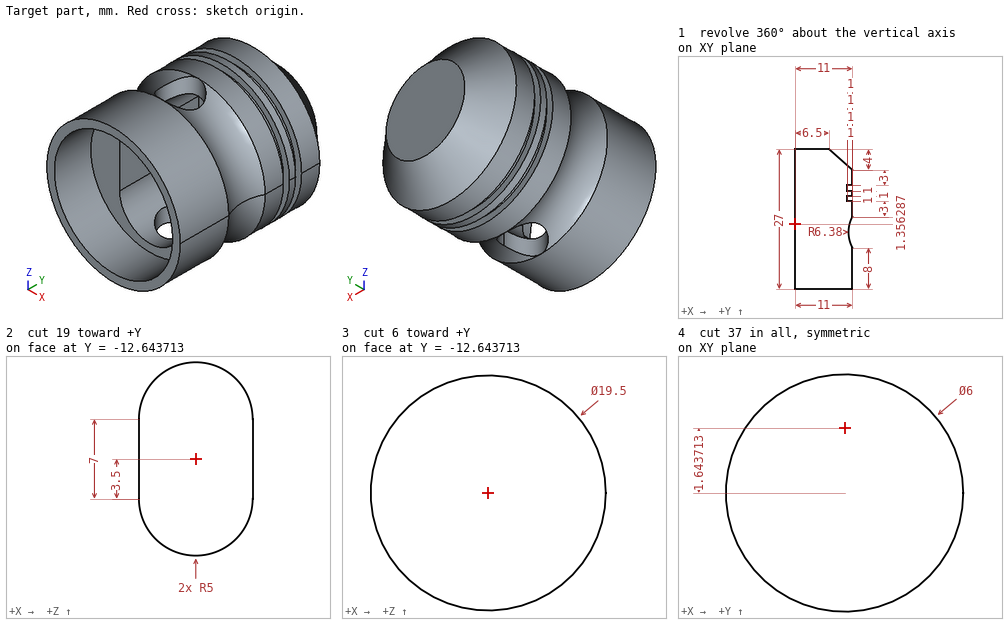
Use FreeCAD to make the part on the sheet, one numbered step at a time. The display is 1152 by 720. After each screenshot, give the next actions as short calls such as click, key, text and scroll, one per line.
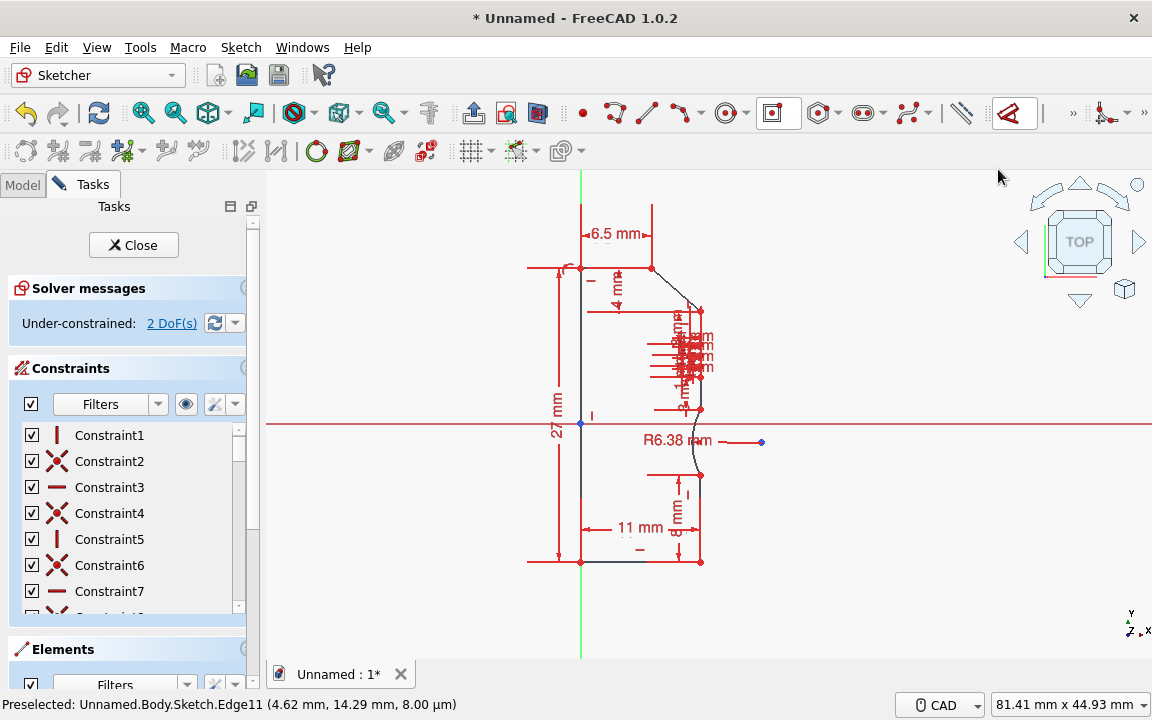
click(701, 410)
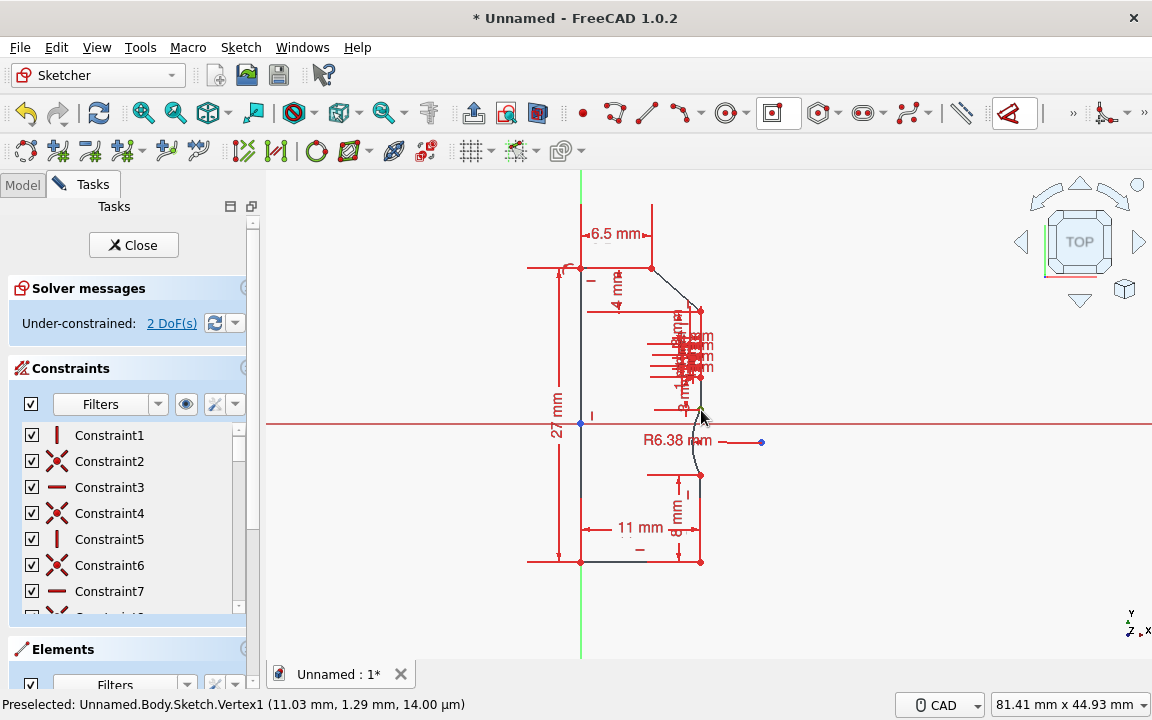
key(l)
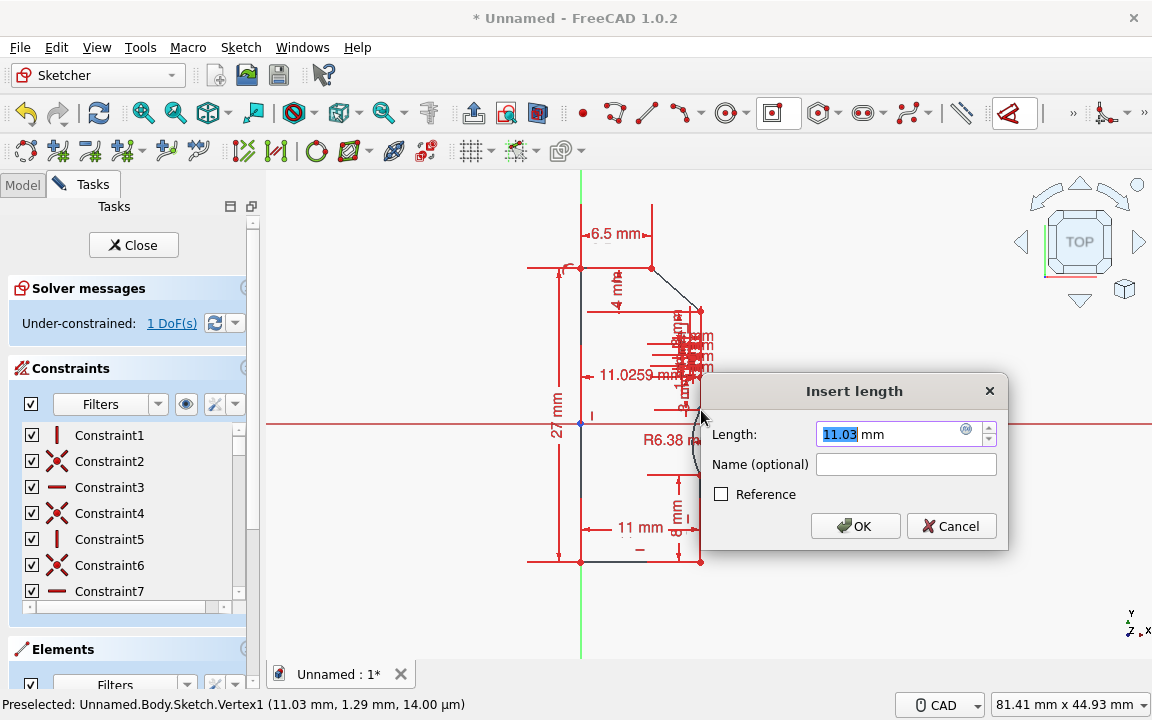
text(11)
key(Return)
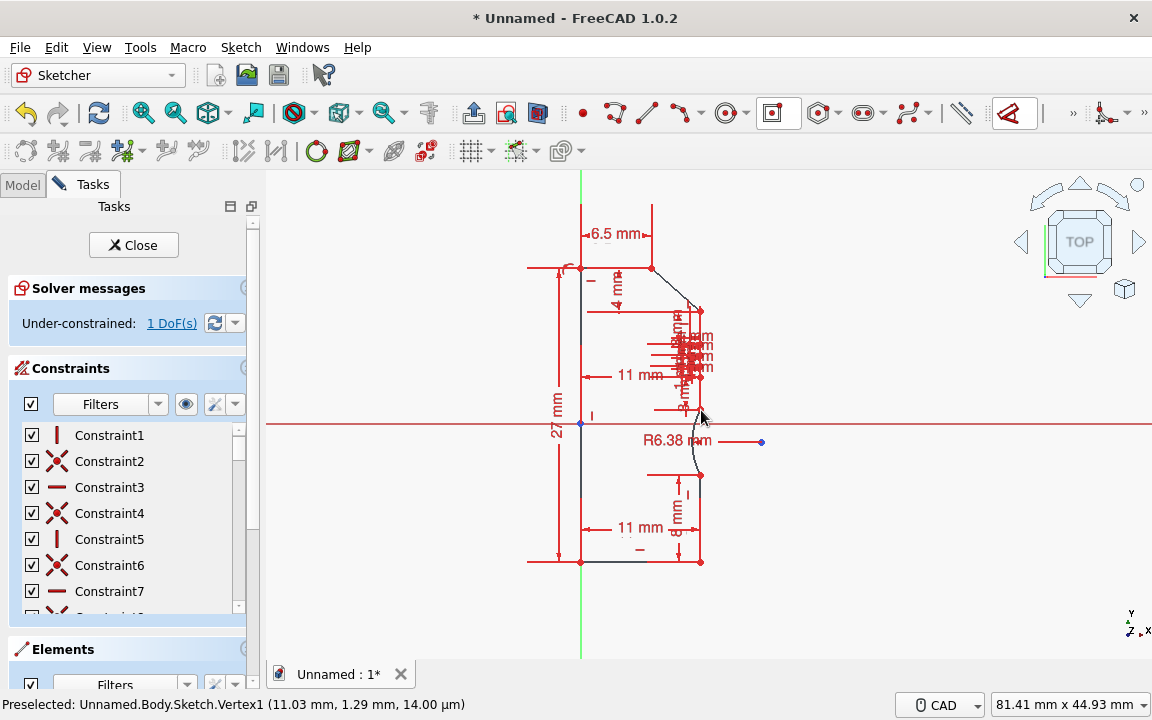
scroll(700, 410, up, 5)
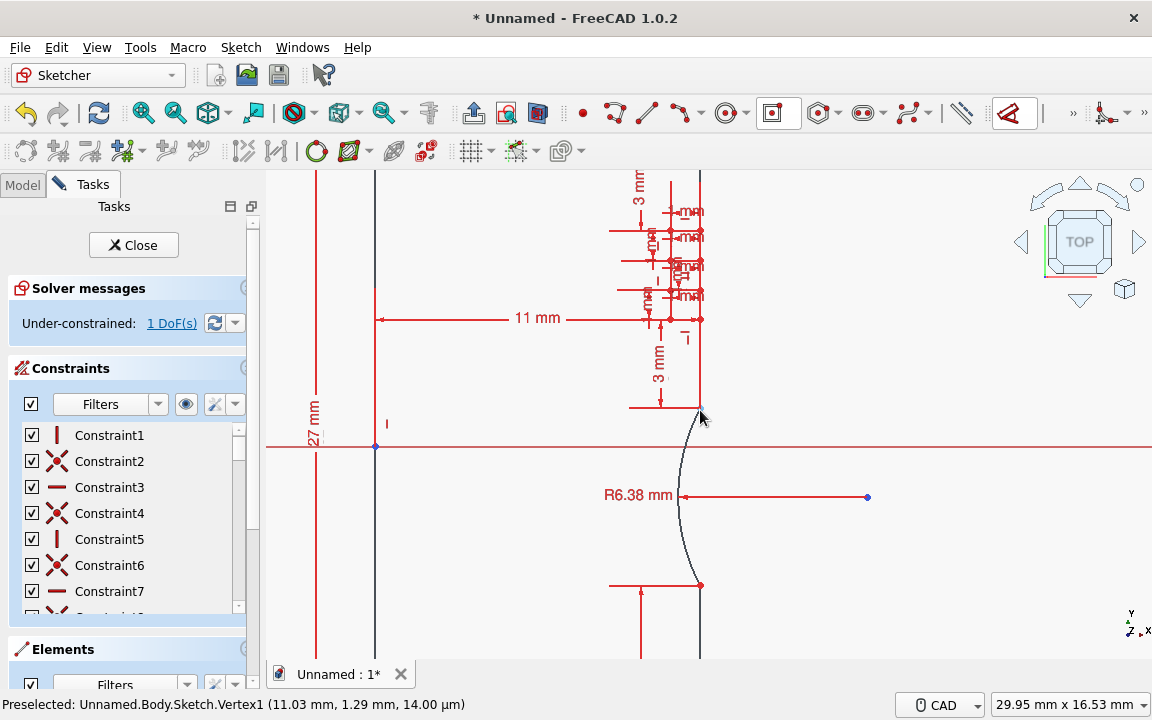
click(700, 408)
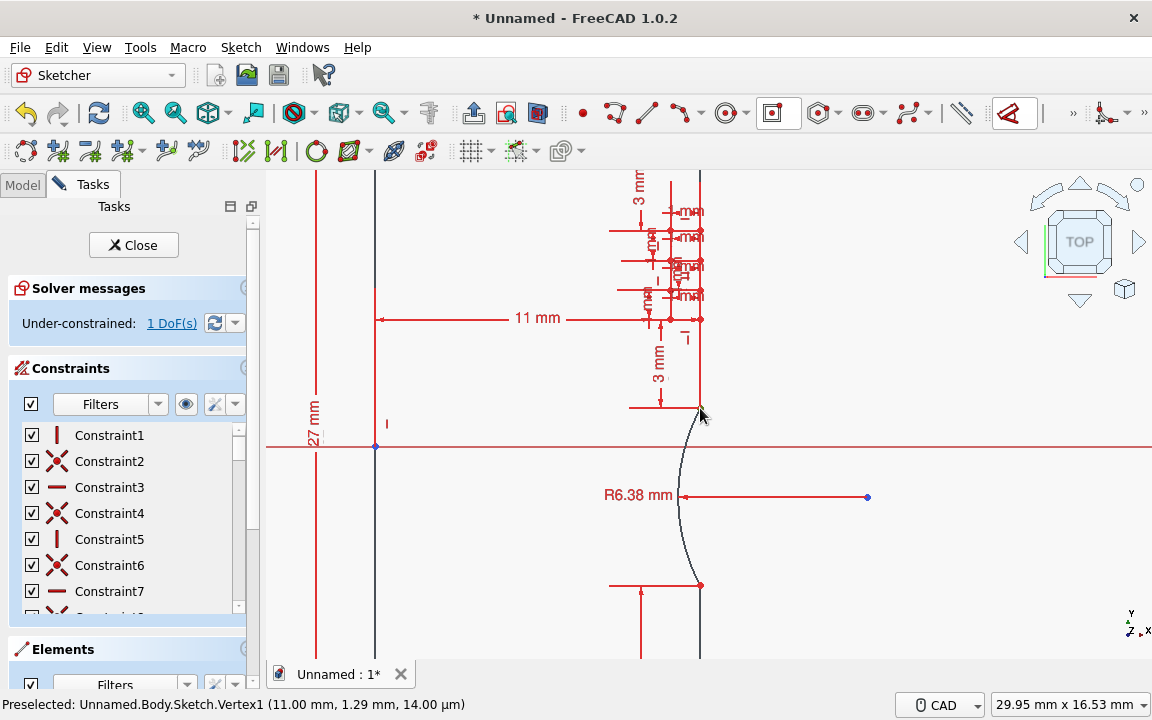
click(1032, 114)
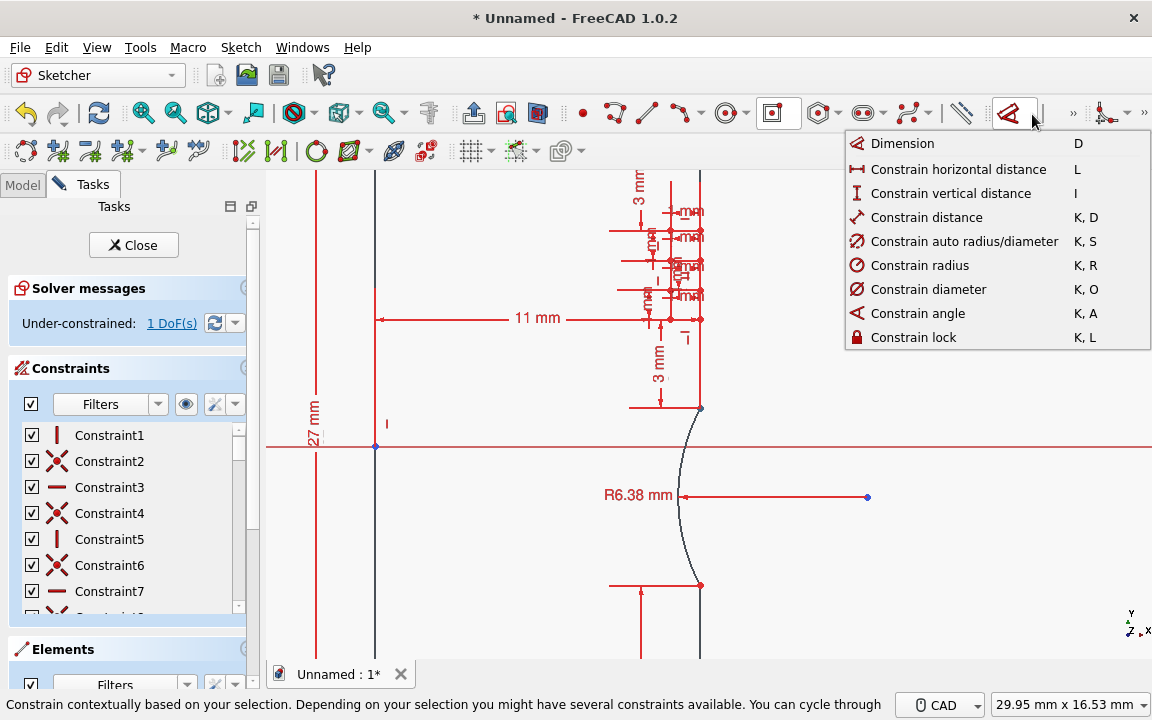
click(998, 193)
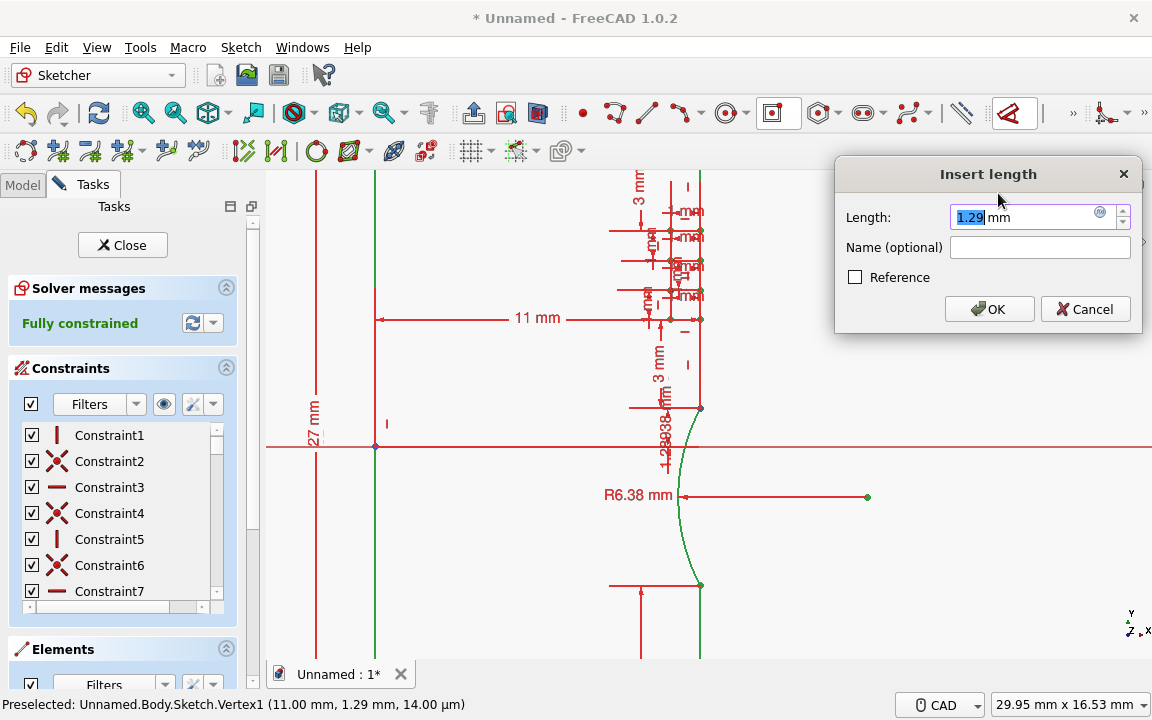
text(1.356287)
key(Return)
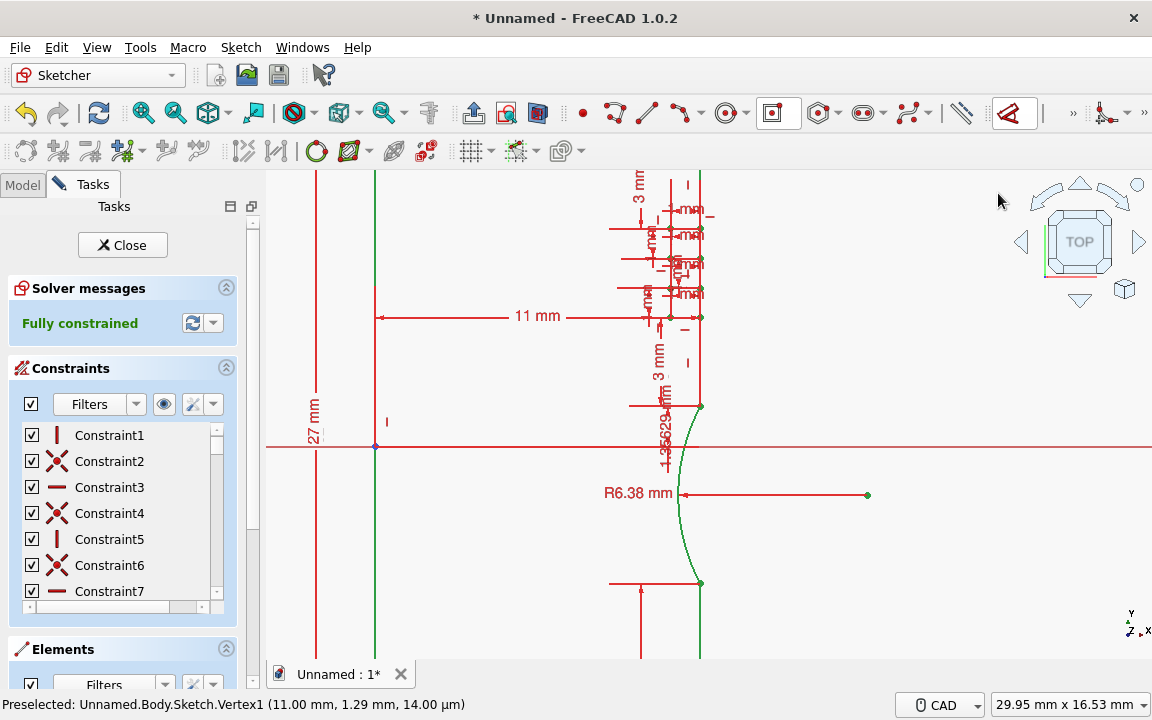
click(123, 245)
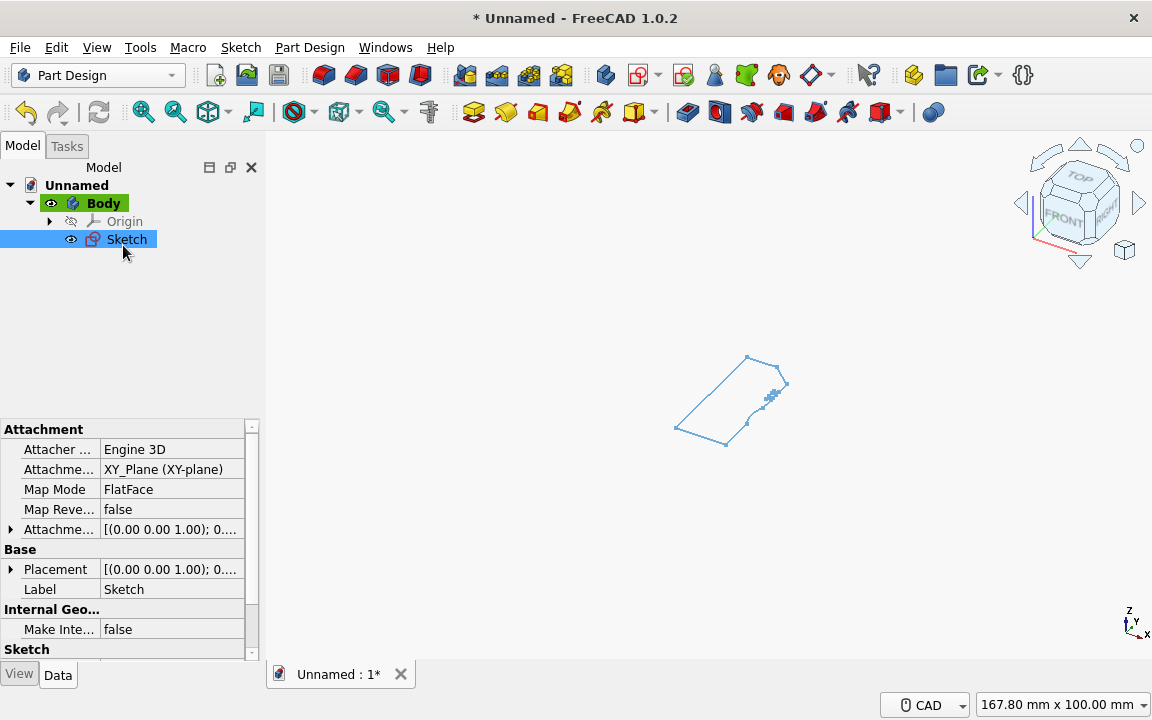
click(506, 112)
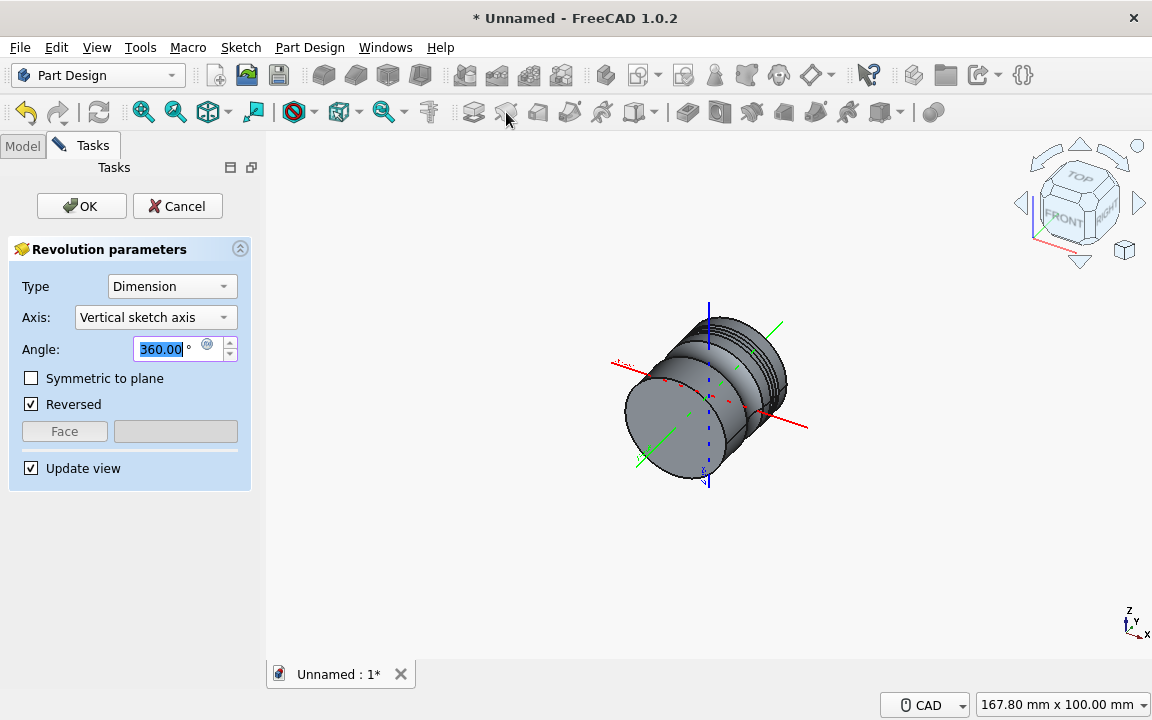
click(82, 206)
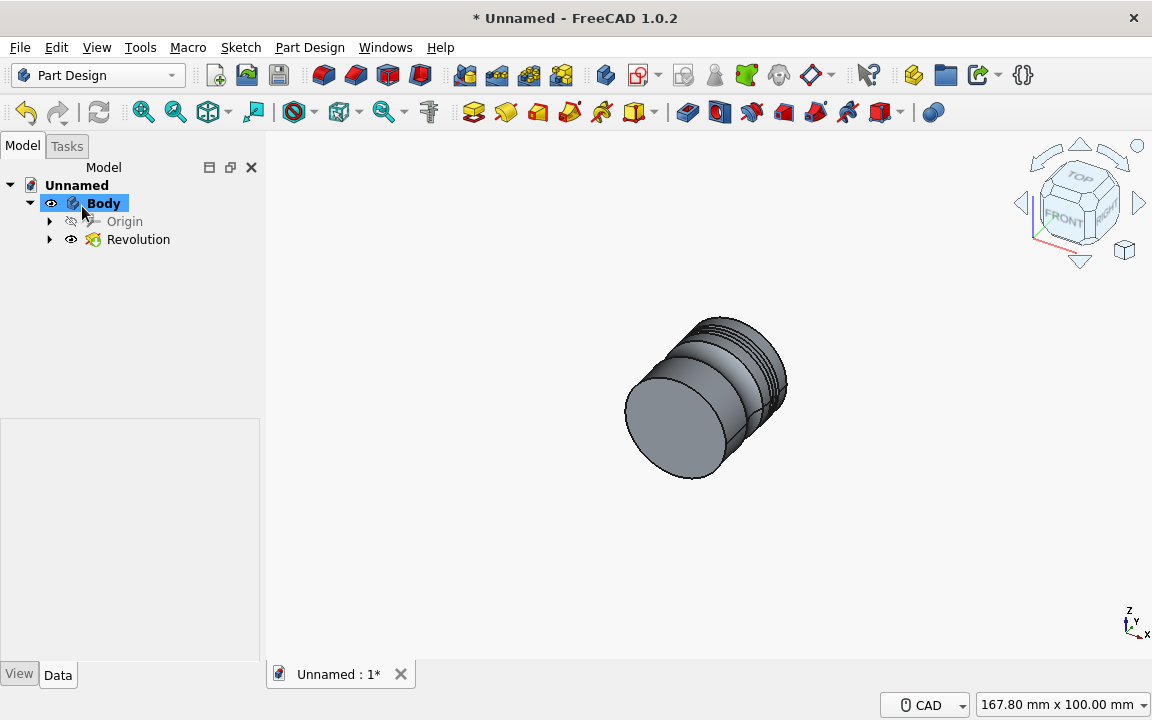
key(v)
key(f)